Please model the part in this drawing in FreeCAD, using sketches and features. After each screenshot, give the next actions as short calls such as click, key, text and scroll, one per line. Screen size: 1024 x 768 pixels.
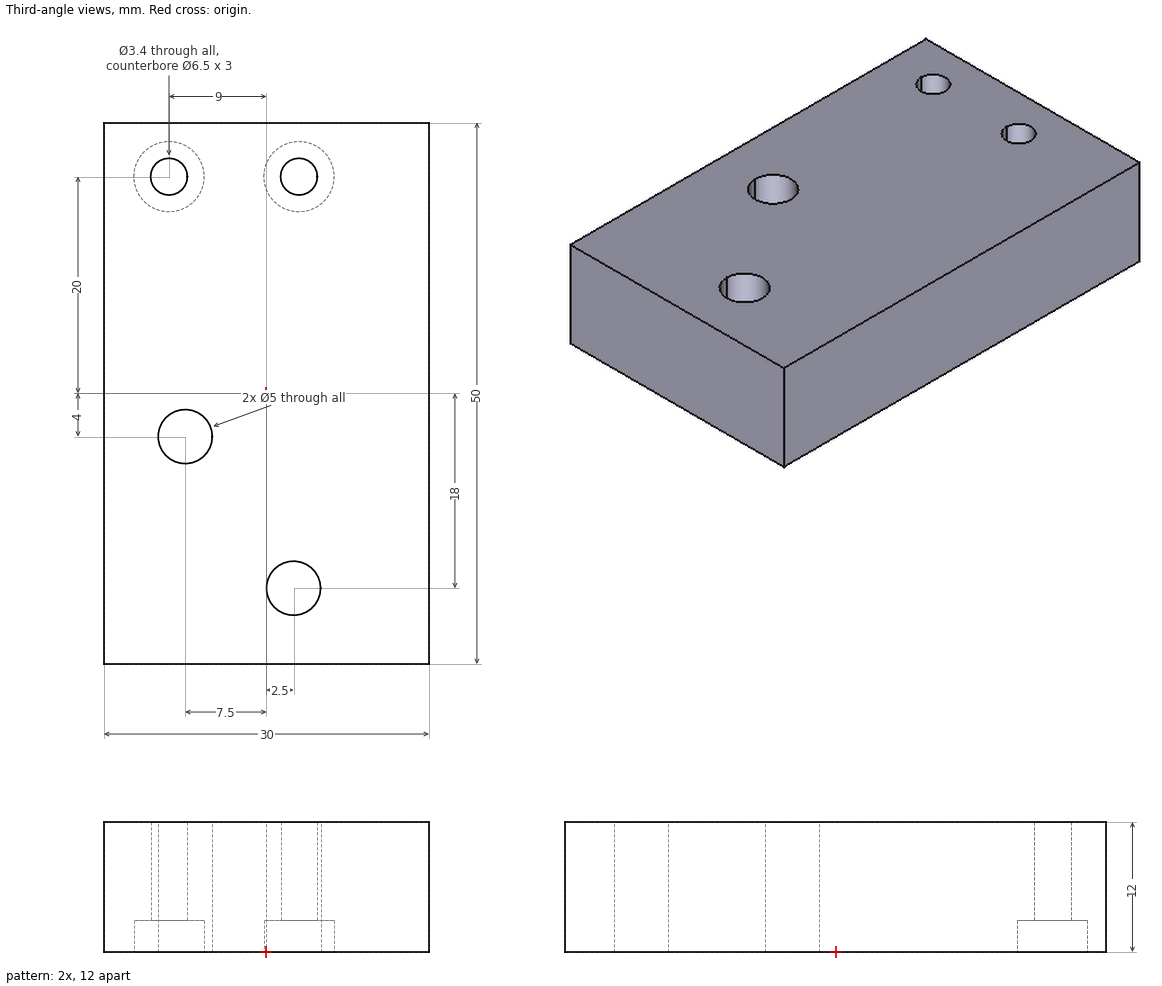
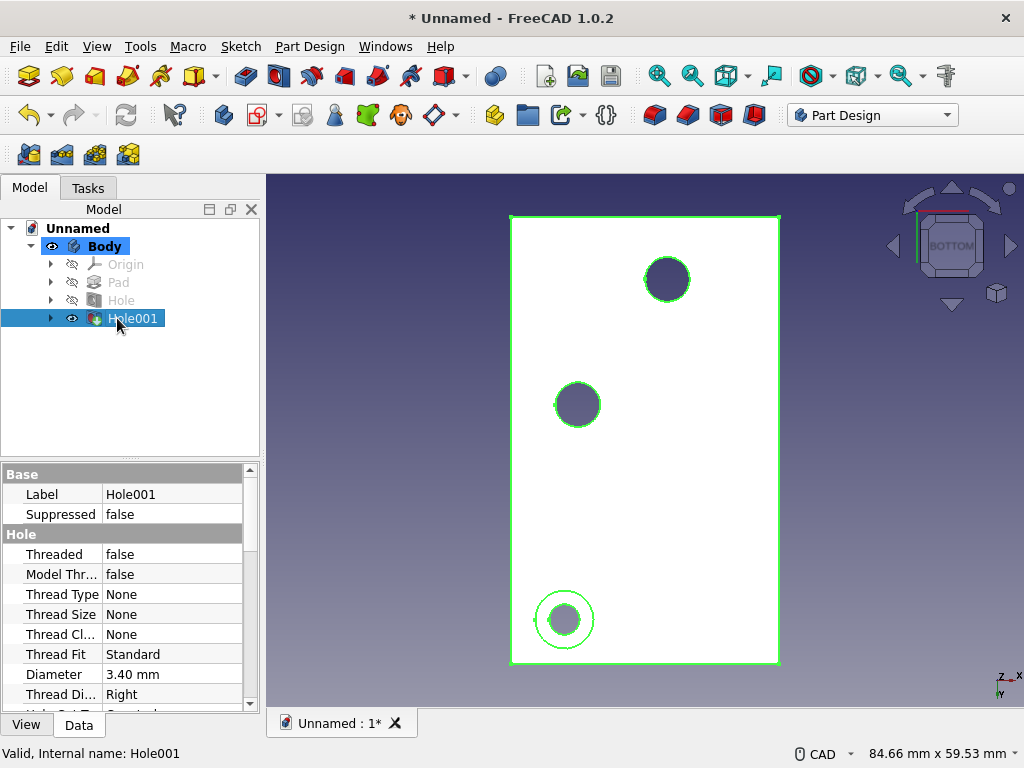
click(62, 154)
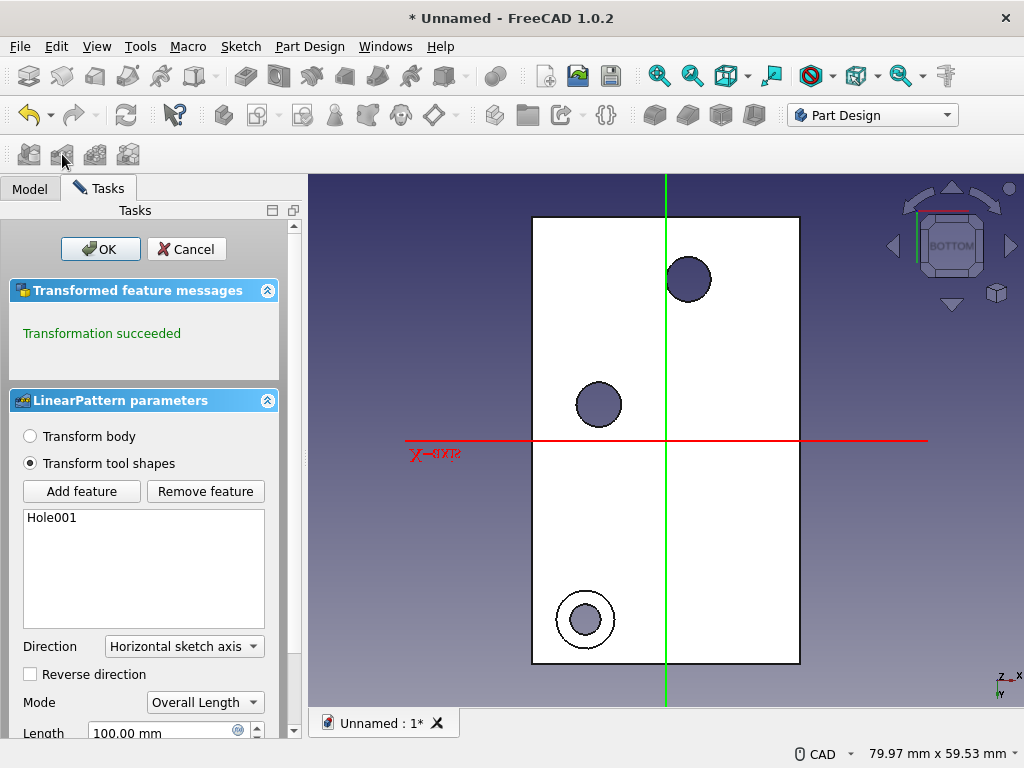
click(185, 646)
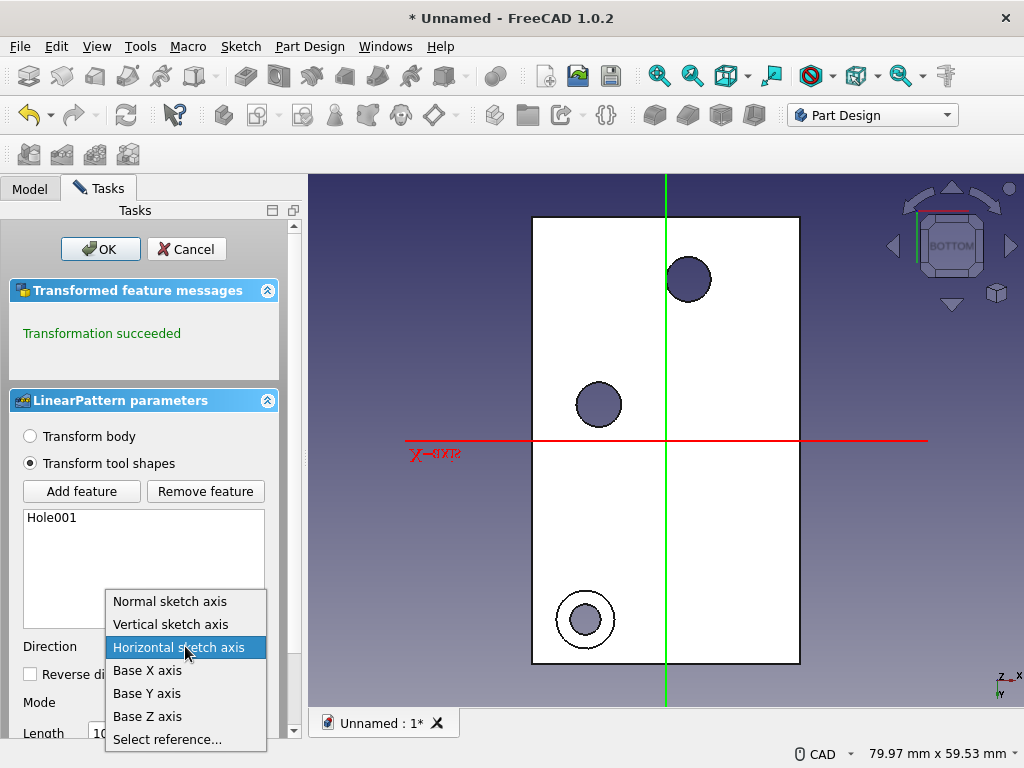
click(184, 670)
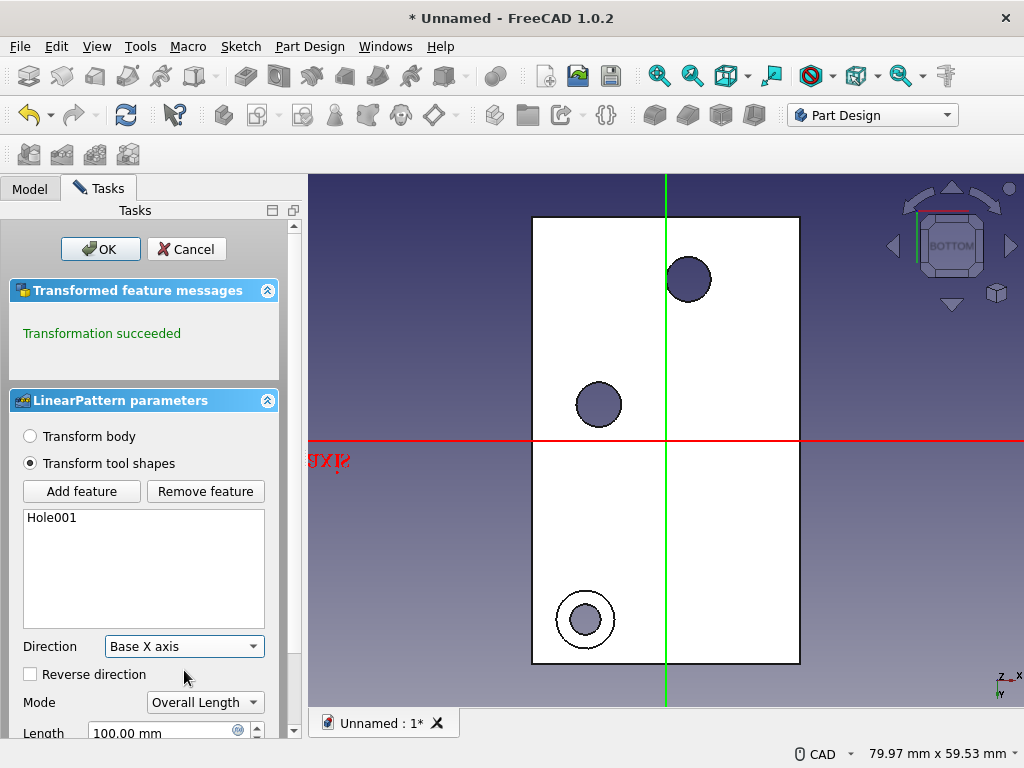
click(206, 702)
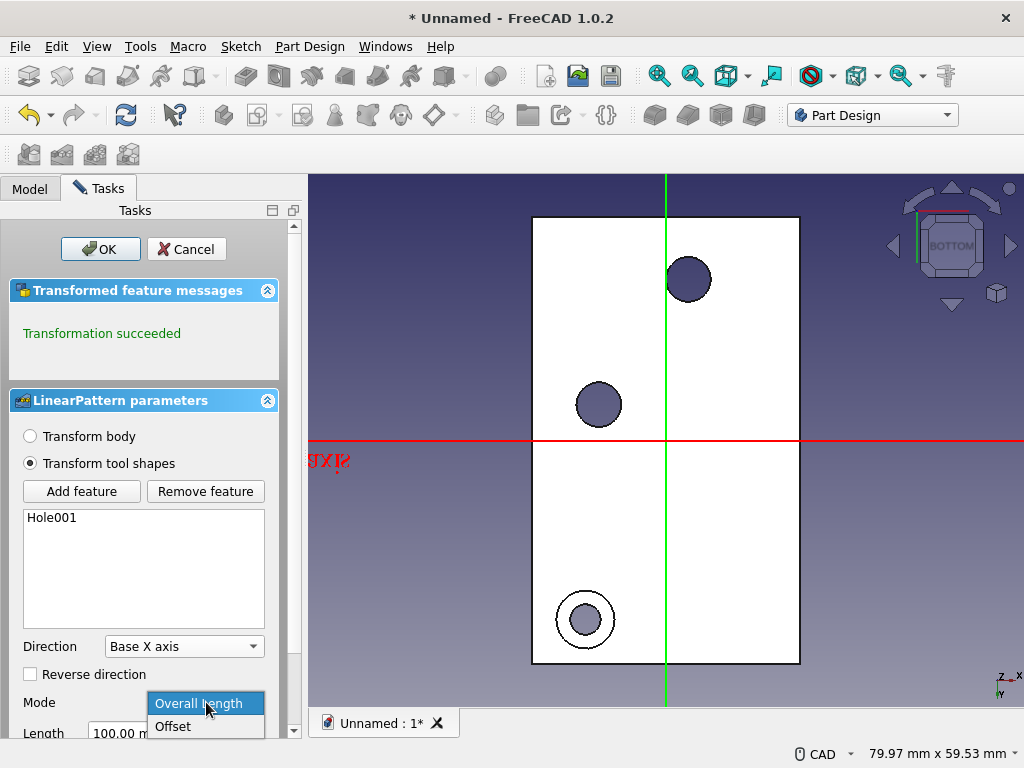
click(204, 726)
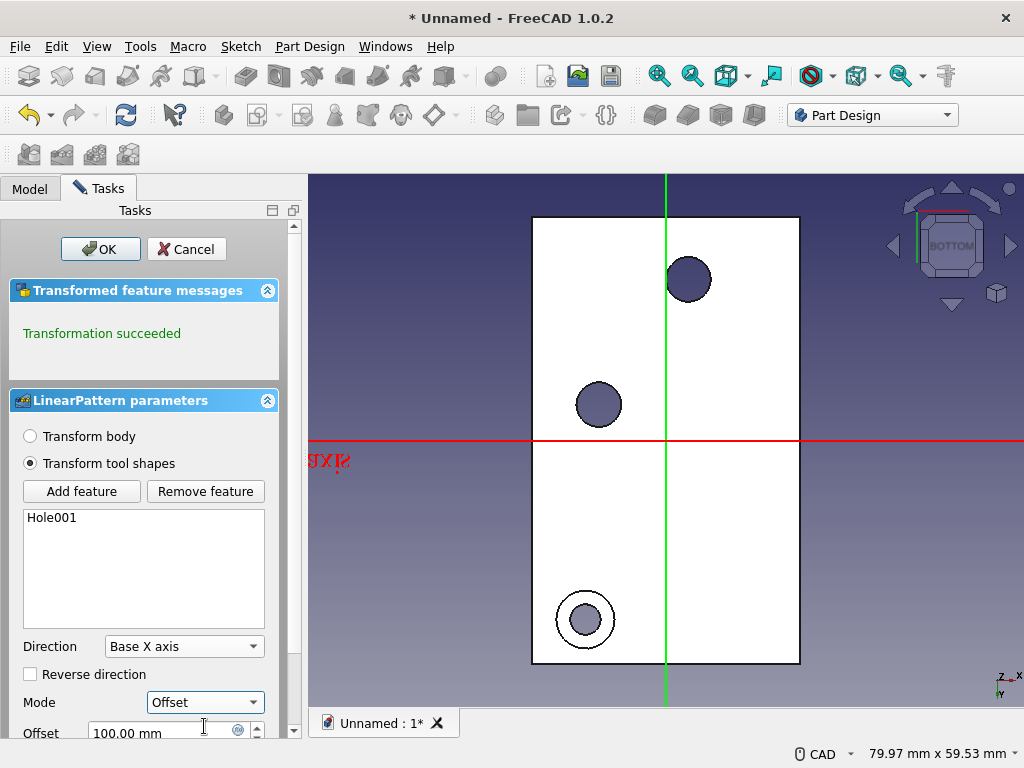
scroll(294, 479, down, 2)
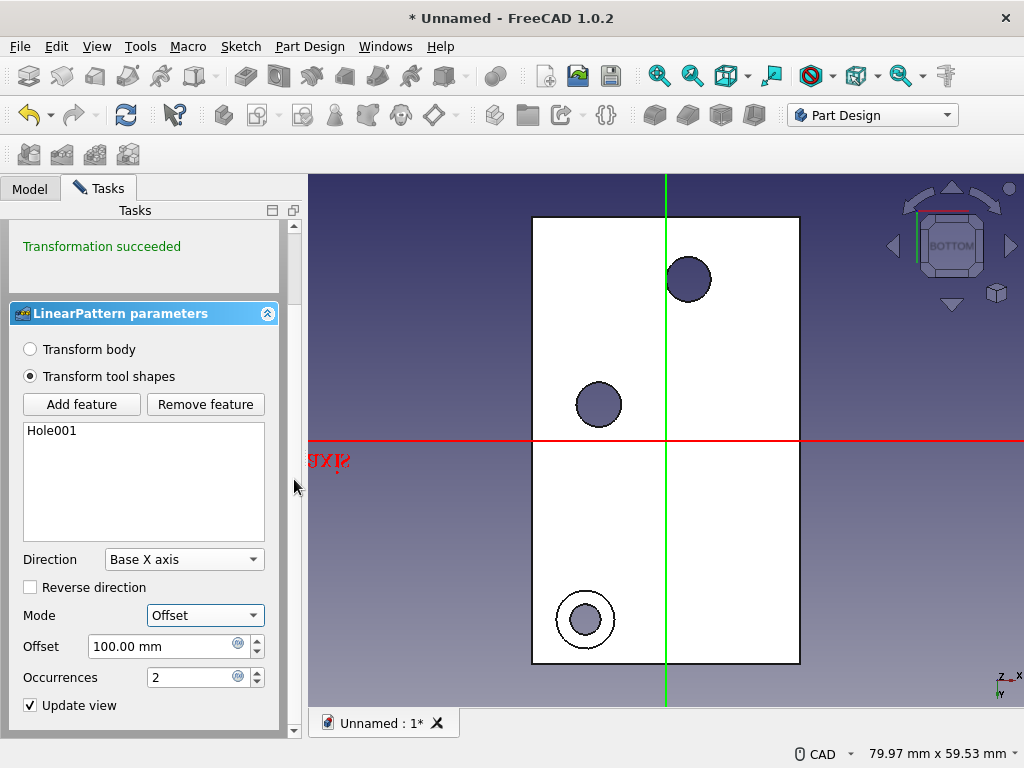
triple_click(170, 646)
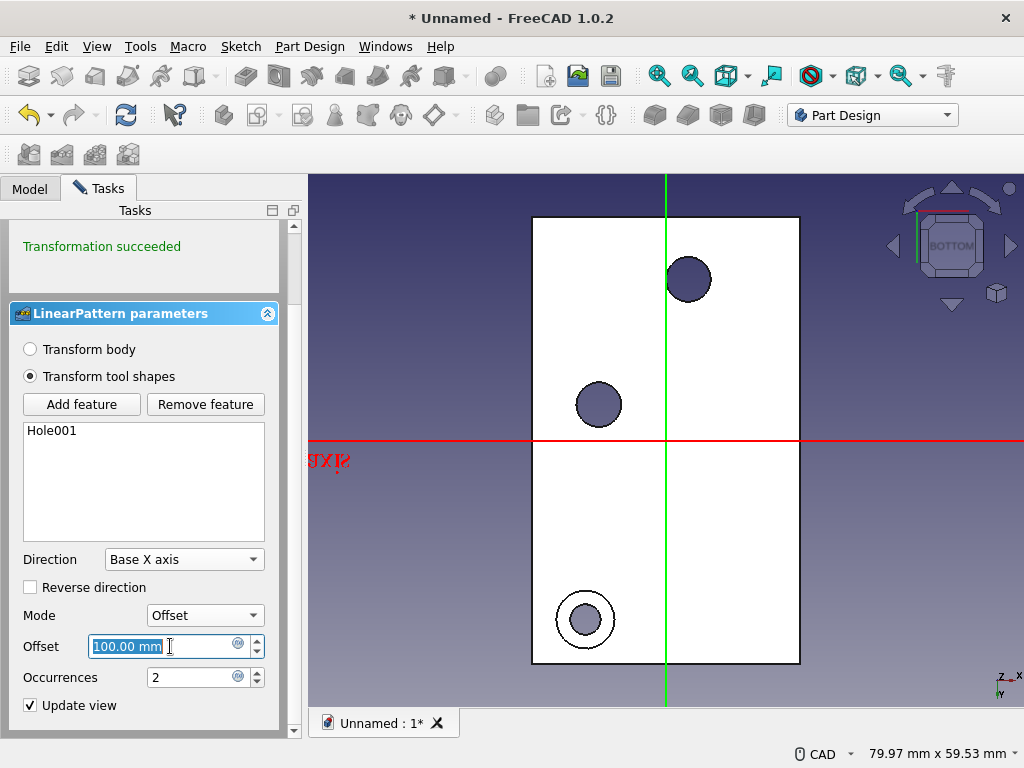
text(12)
key(Tab)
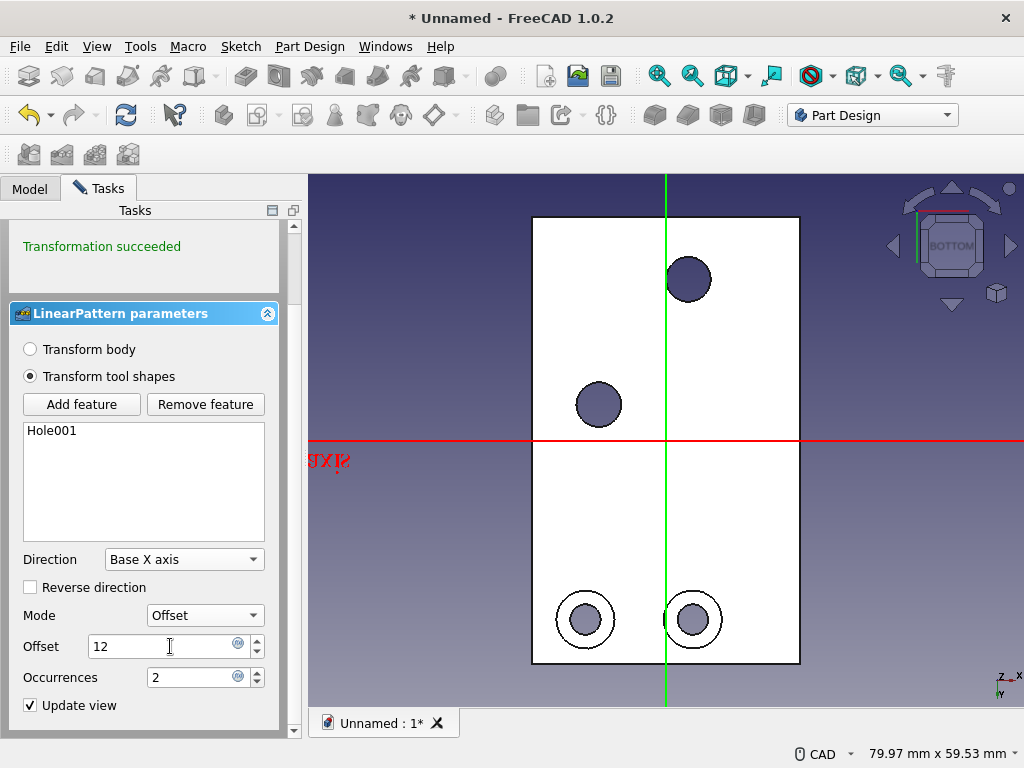
triple_click(199, 678)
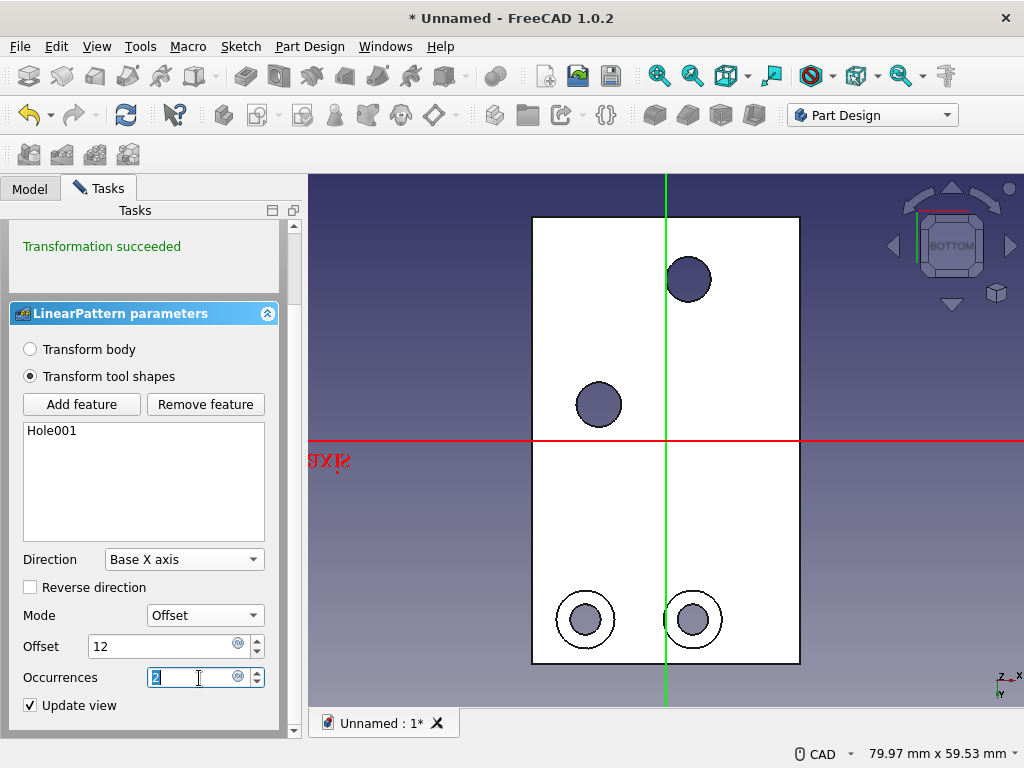
text(2)
key(Tab)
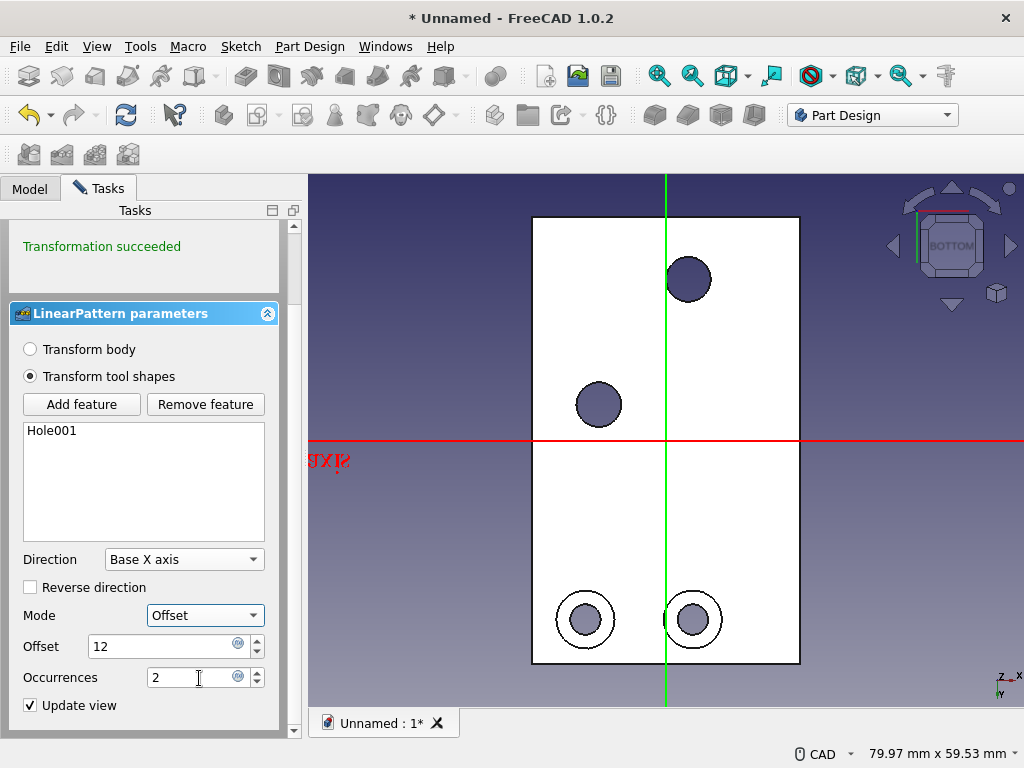
scroll(294, 479, up, 3)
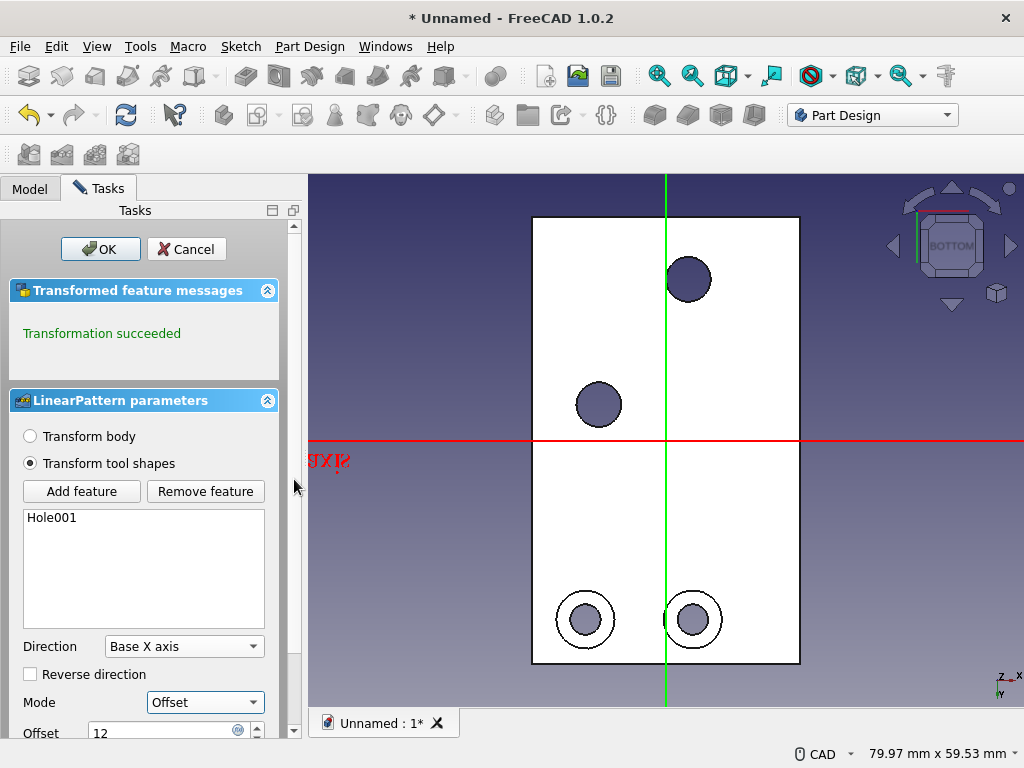
click(101, 249)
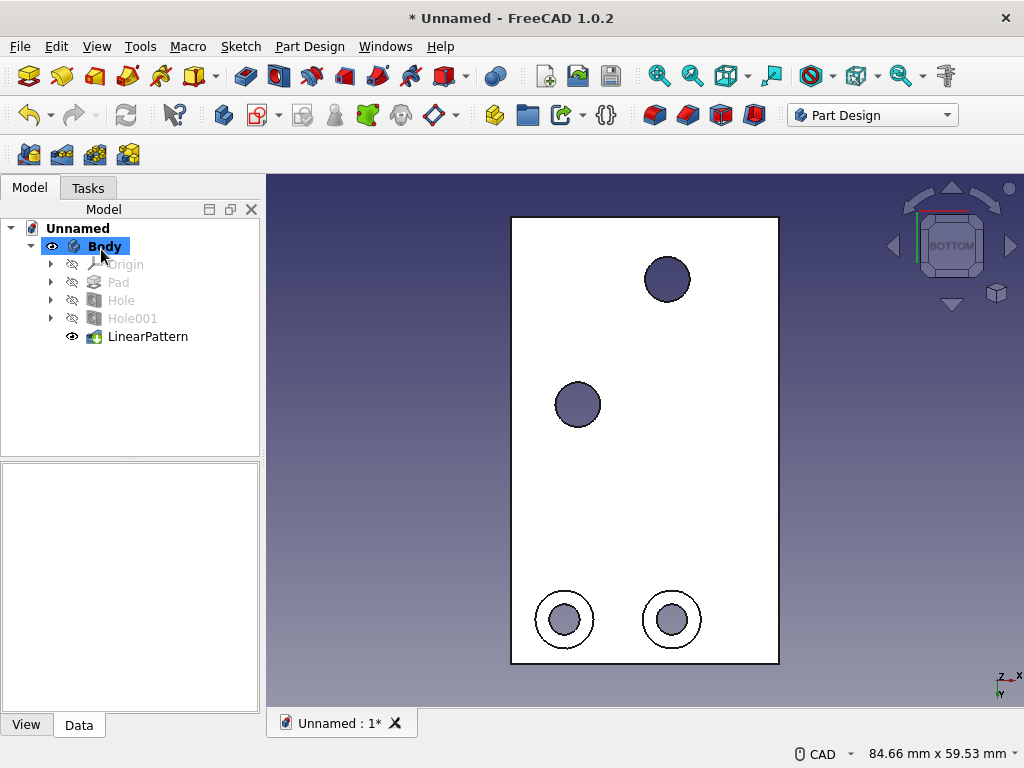
key(0)